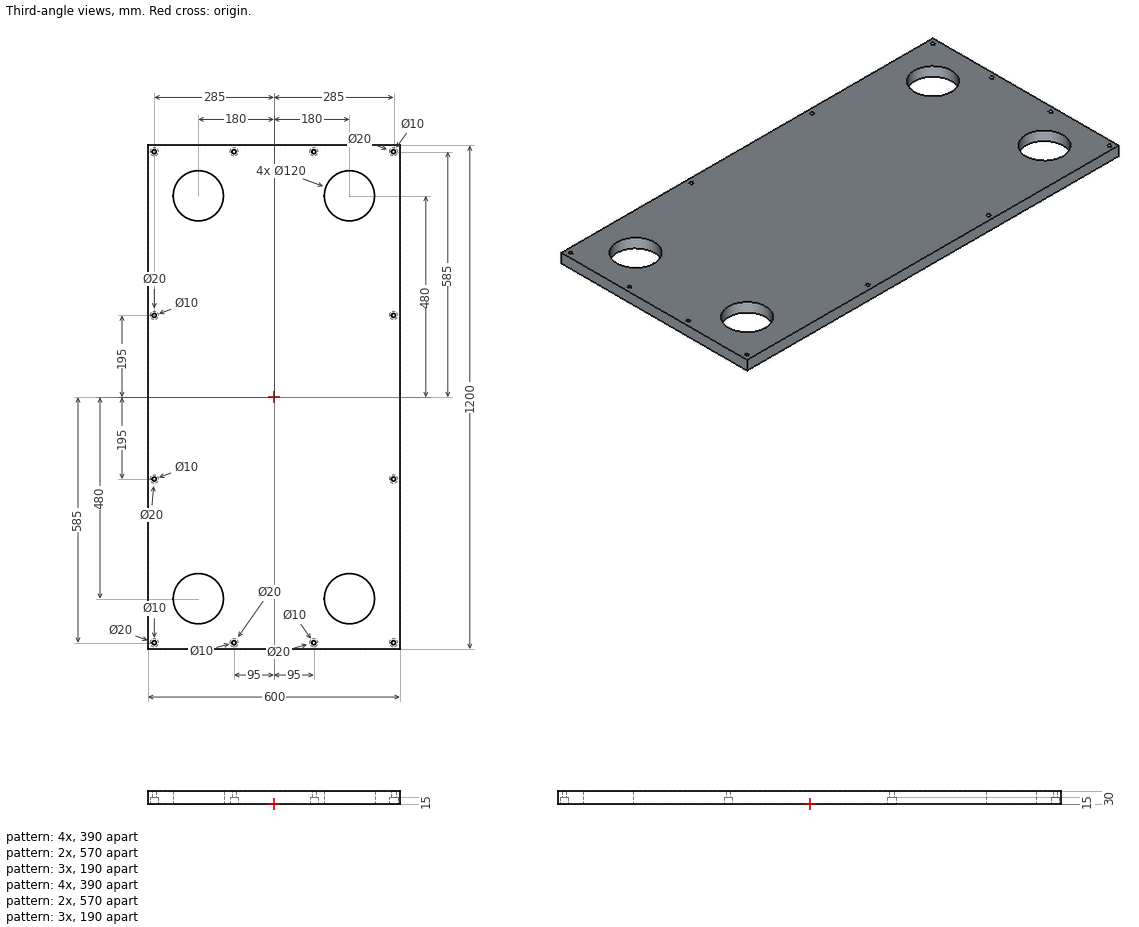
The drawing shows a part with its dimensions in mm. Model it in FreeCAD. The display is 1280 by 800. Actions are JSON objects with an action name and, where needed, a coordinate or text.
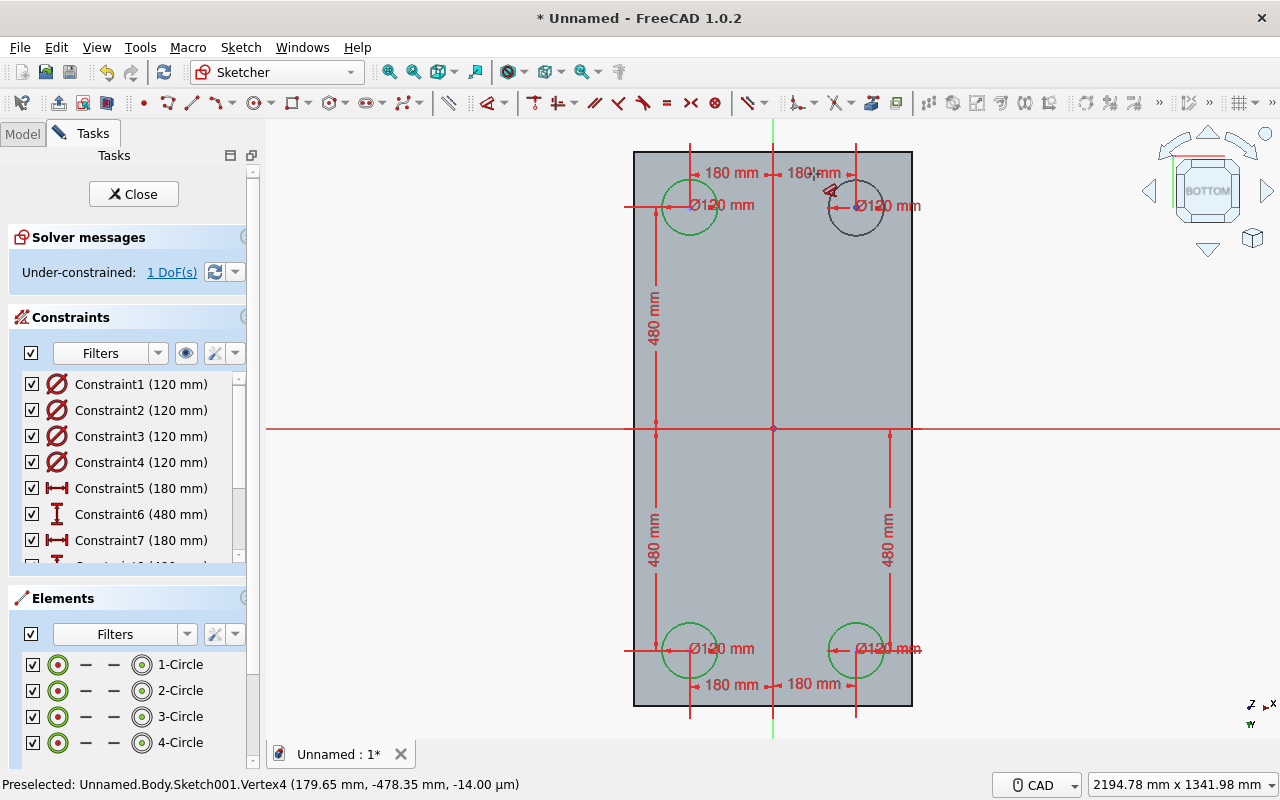
{"action": "left_click", "coordinate": [856, 208]}
{"action": "left_click", "coordinate": [890, 318]}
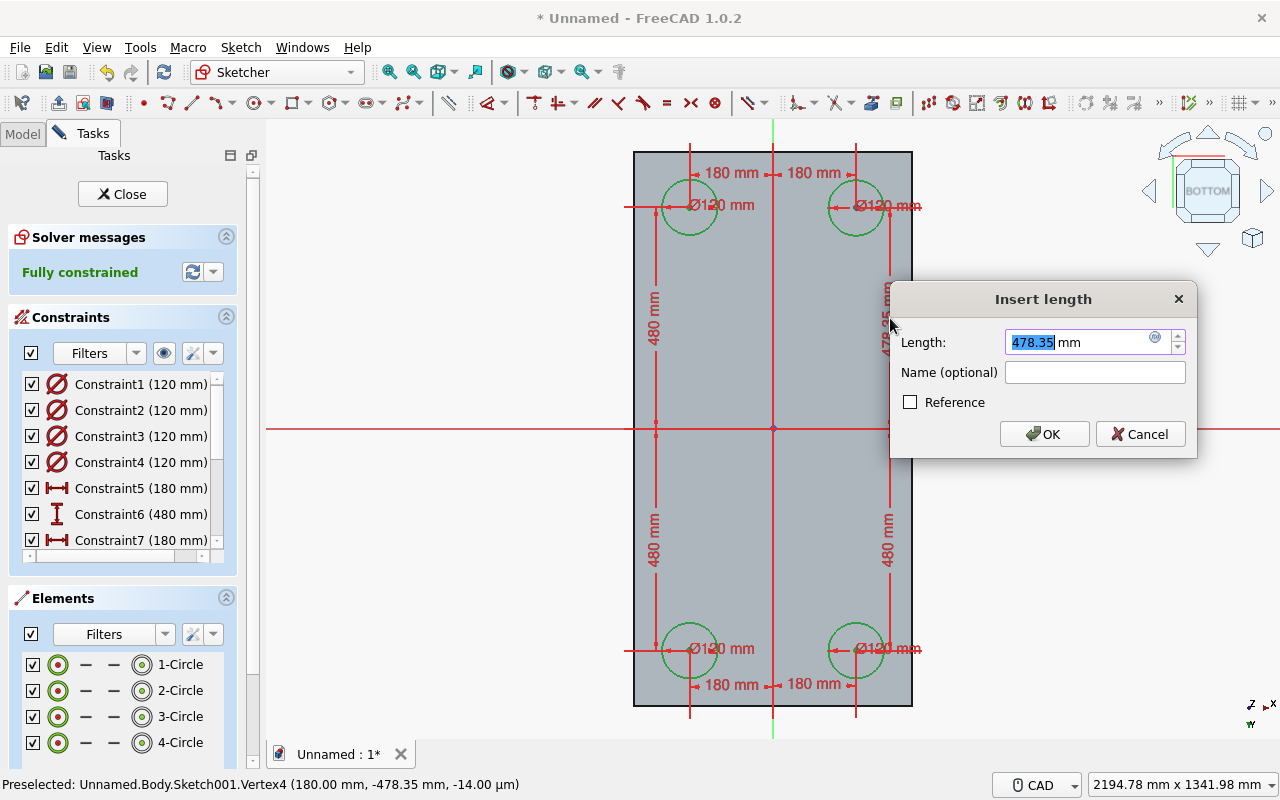
{"action": "type", "text": "480"}
{"action": "key", "text": "Return"}
{"action": "key", "text": "Escape"}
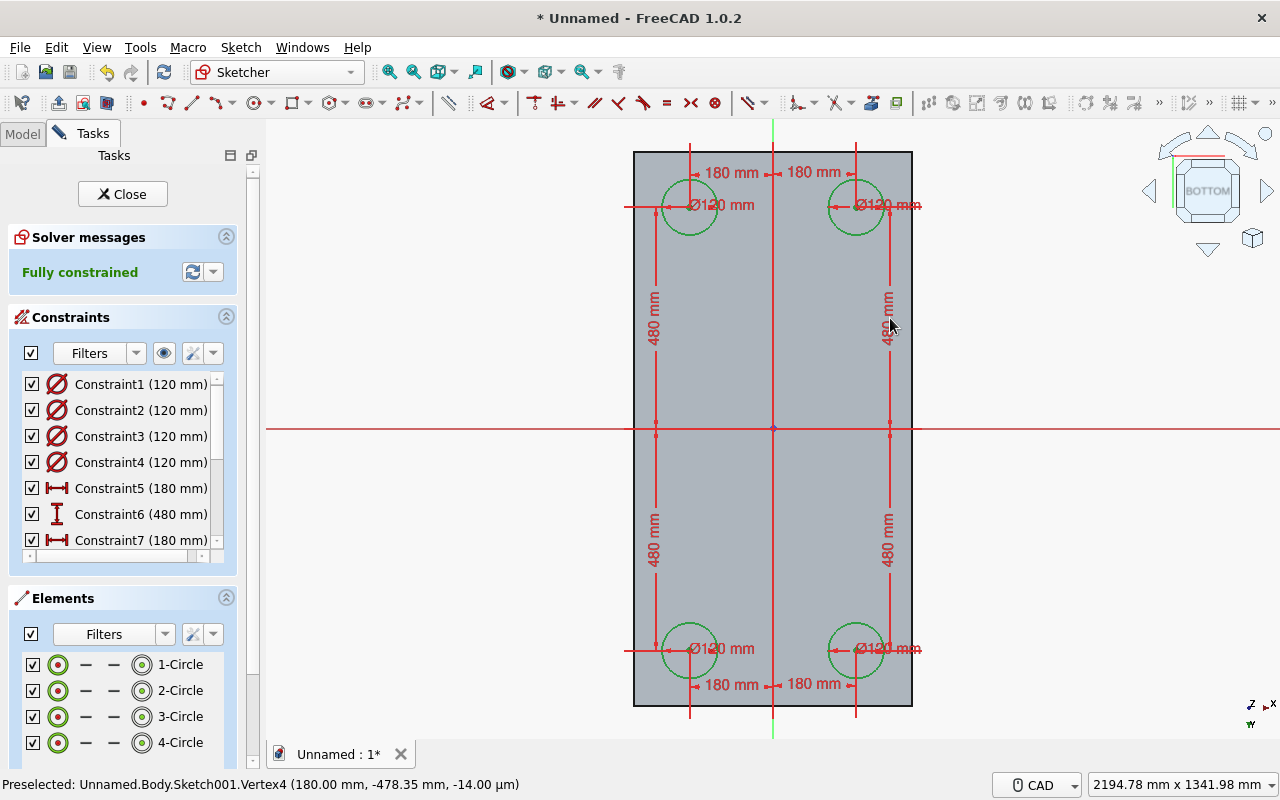
{"action": "left_click", "coordinate": [123, 194]}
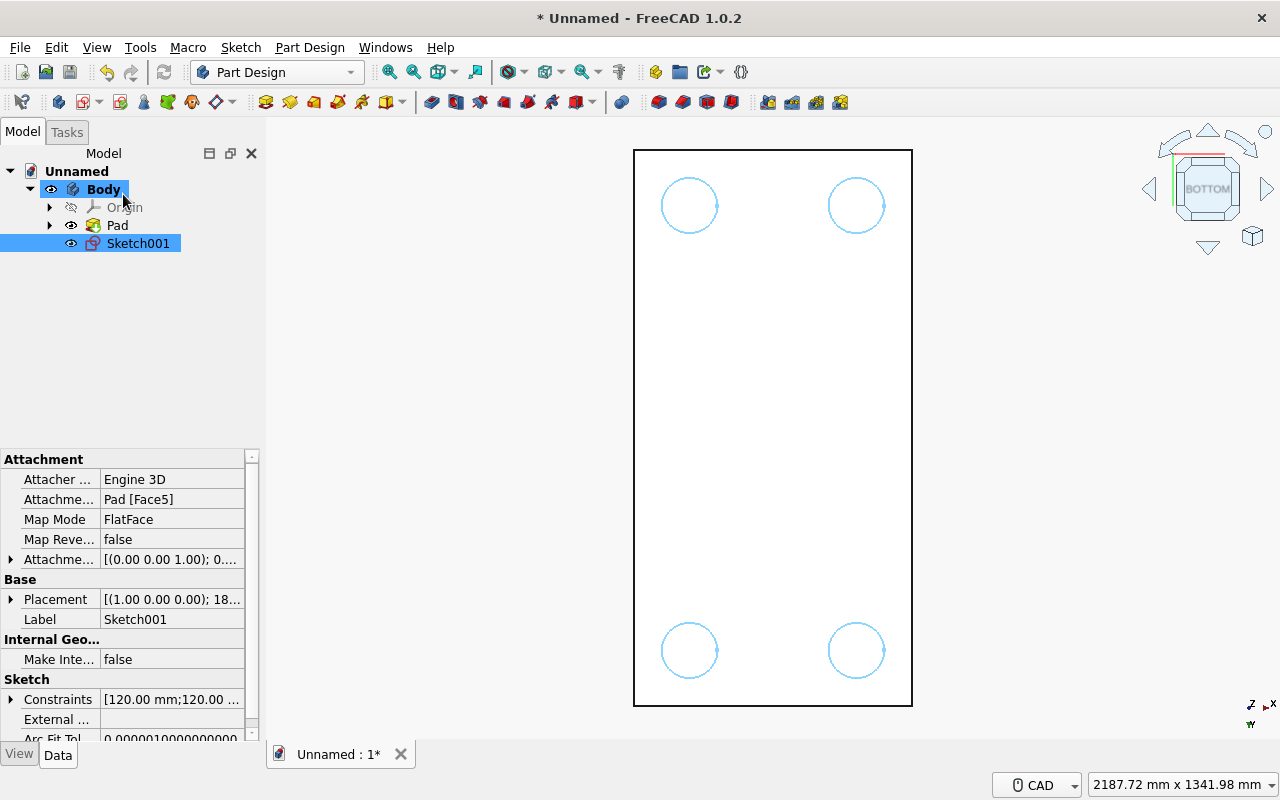
{"action": "left_click", "coordinate": [432, 102]}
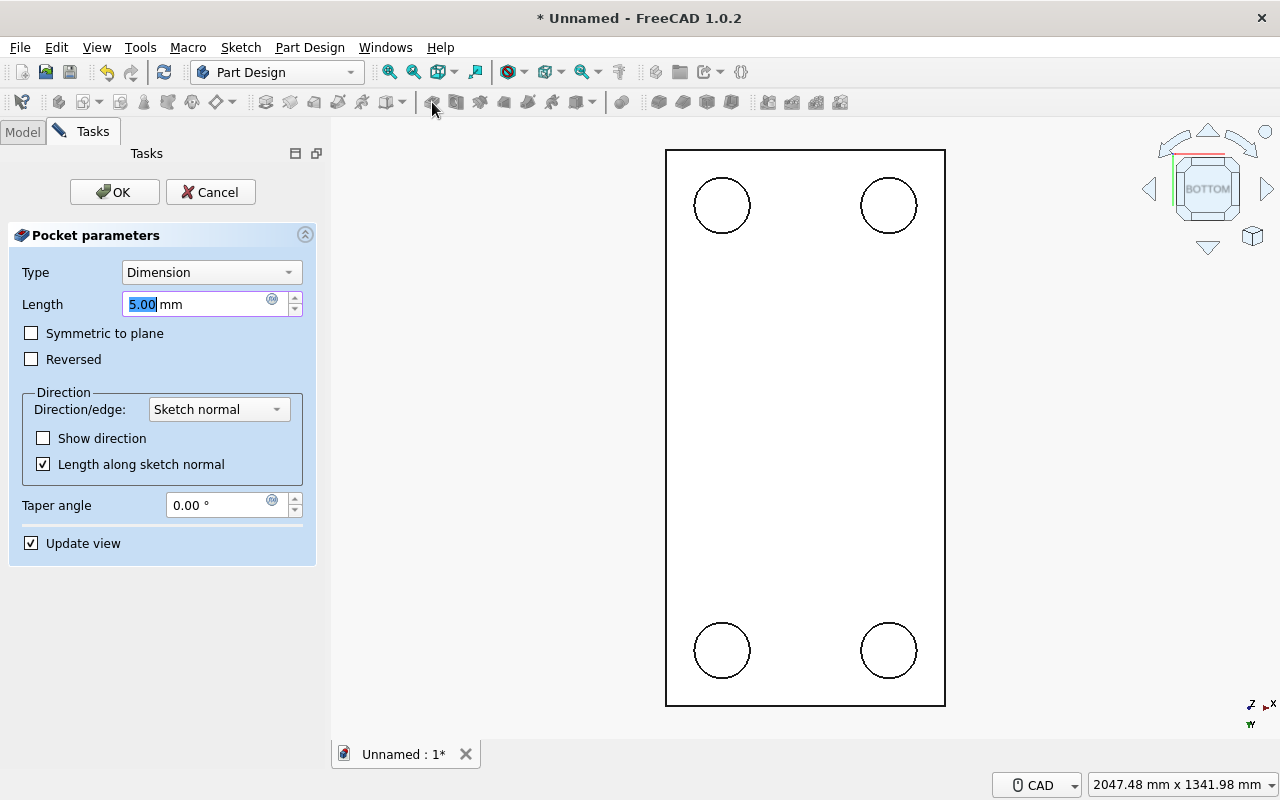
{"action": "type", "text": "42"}
{"action": "key", "text": "Tab"}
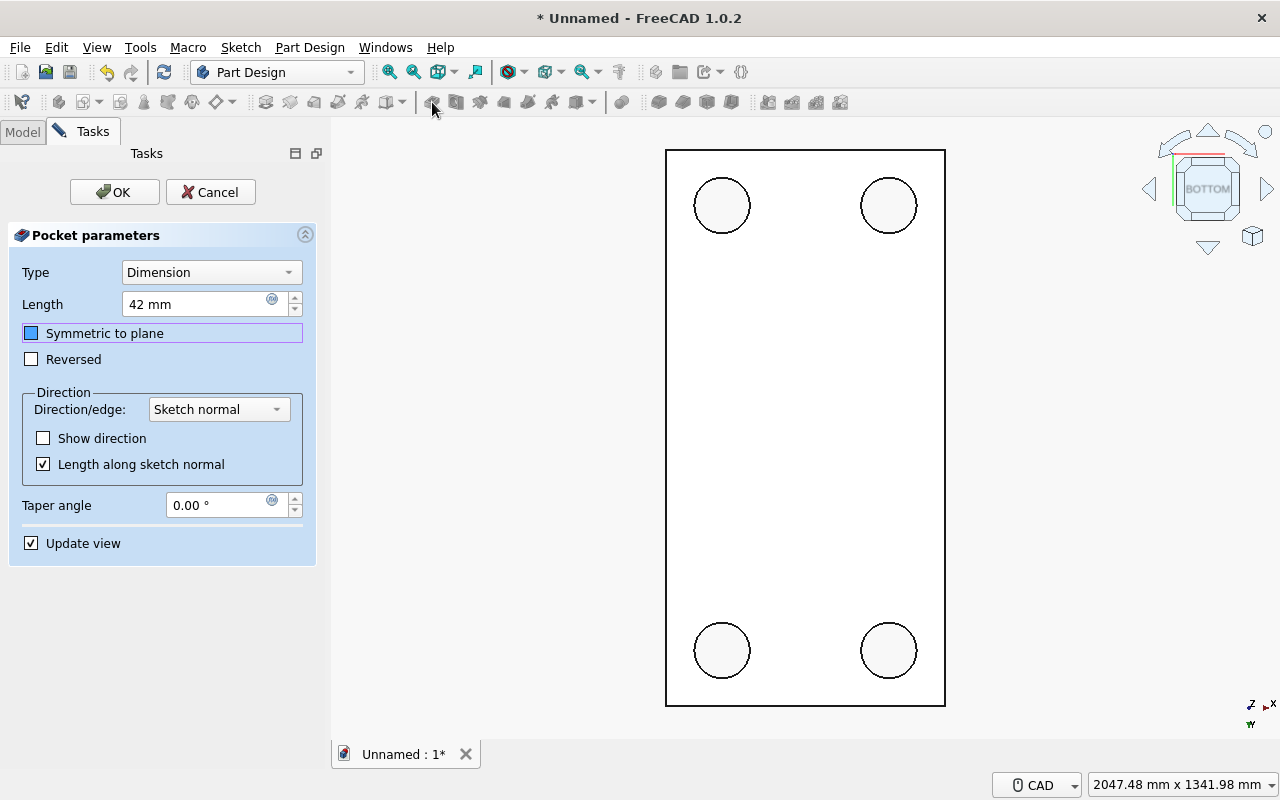
{"action": "left_click", "coordinate": [115, 192]}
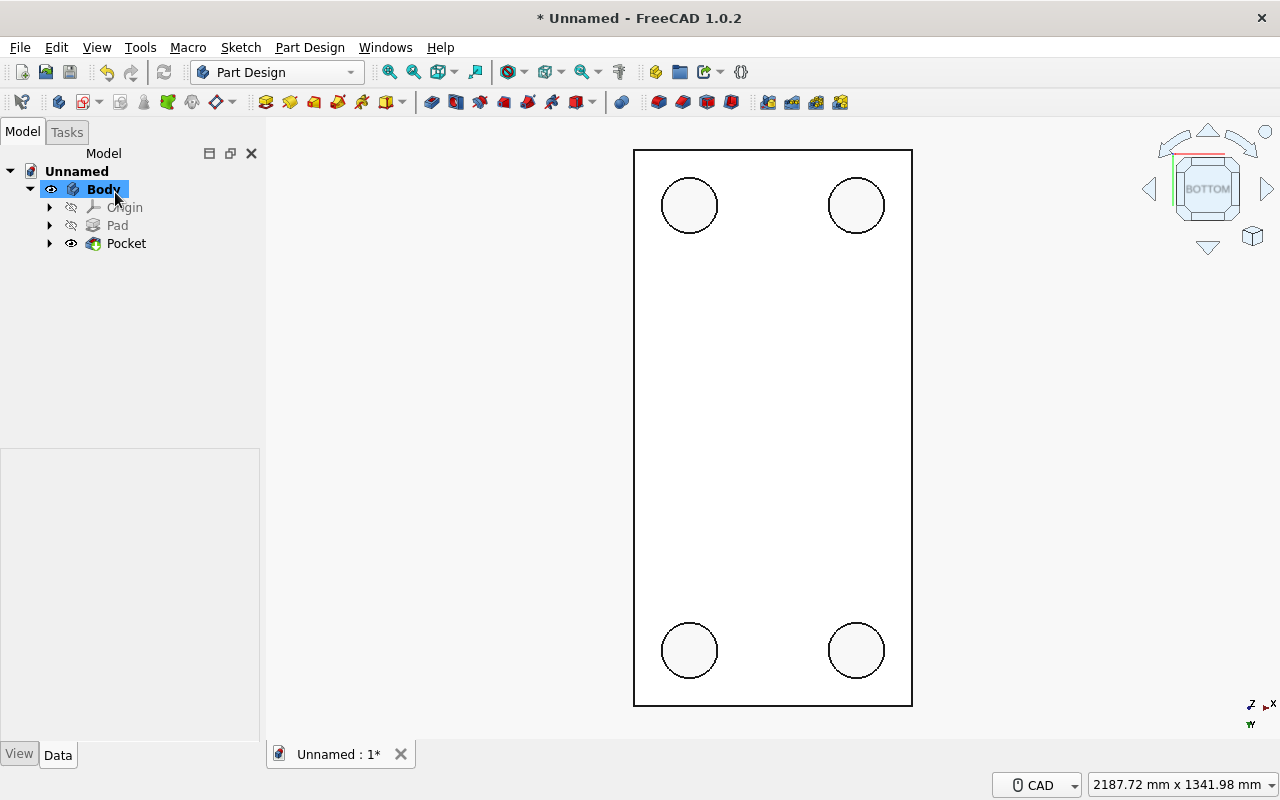
{"action": "left_click", "coordinate": [84, 102]}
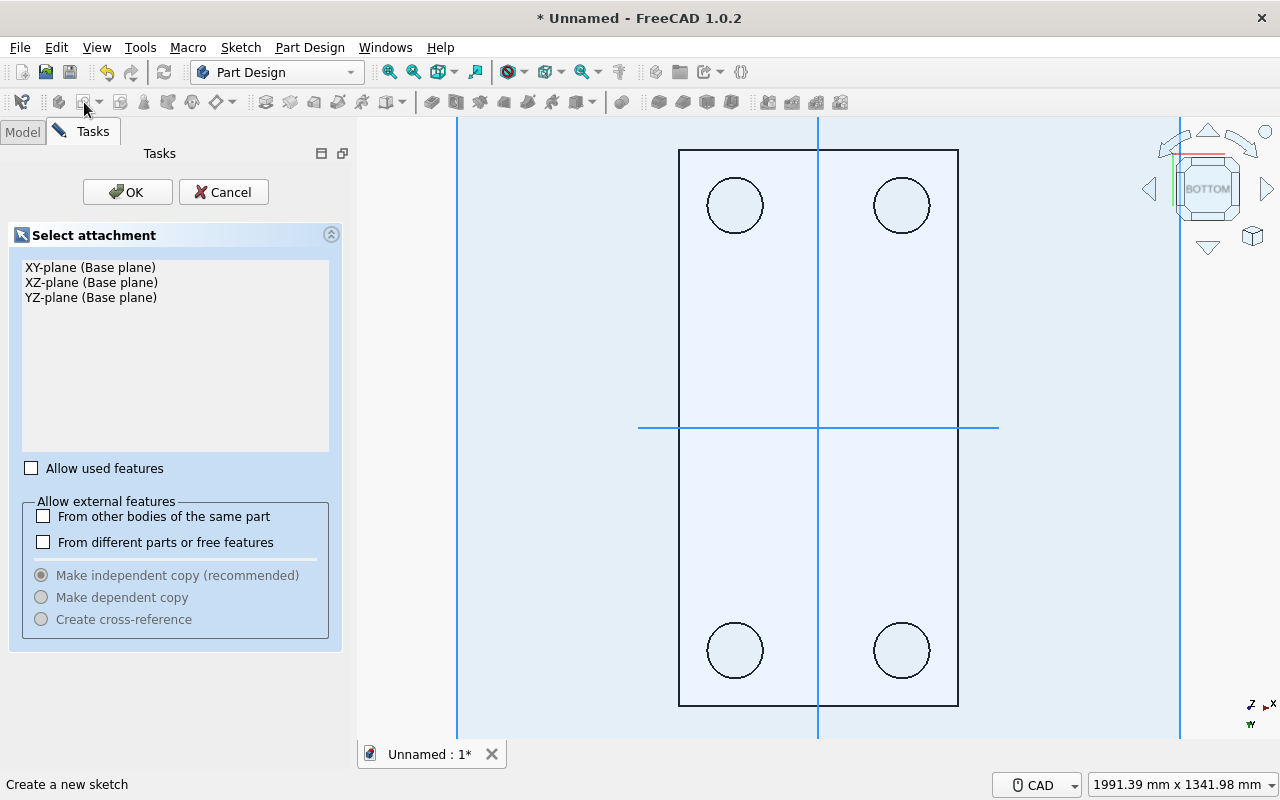
{"action": "left_click", "coordinate": [82, 268]}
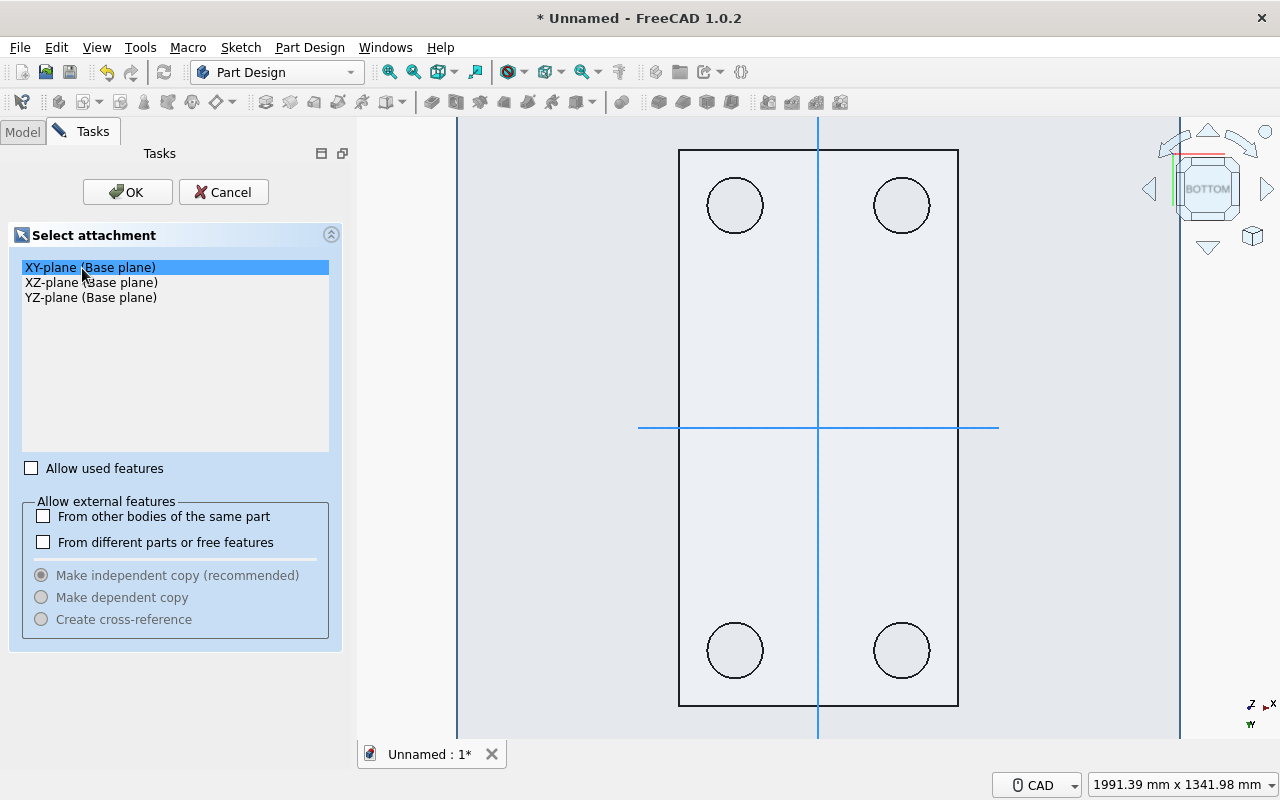
{"action": "left_click", "coordinate": [128, 192]}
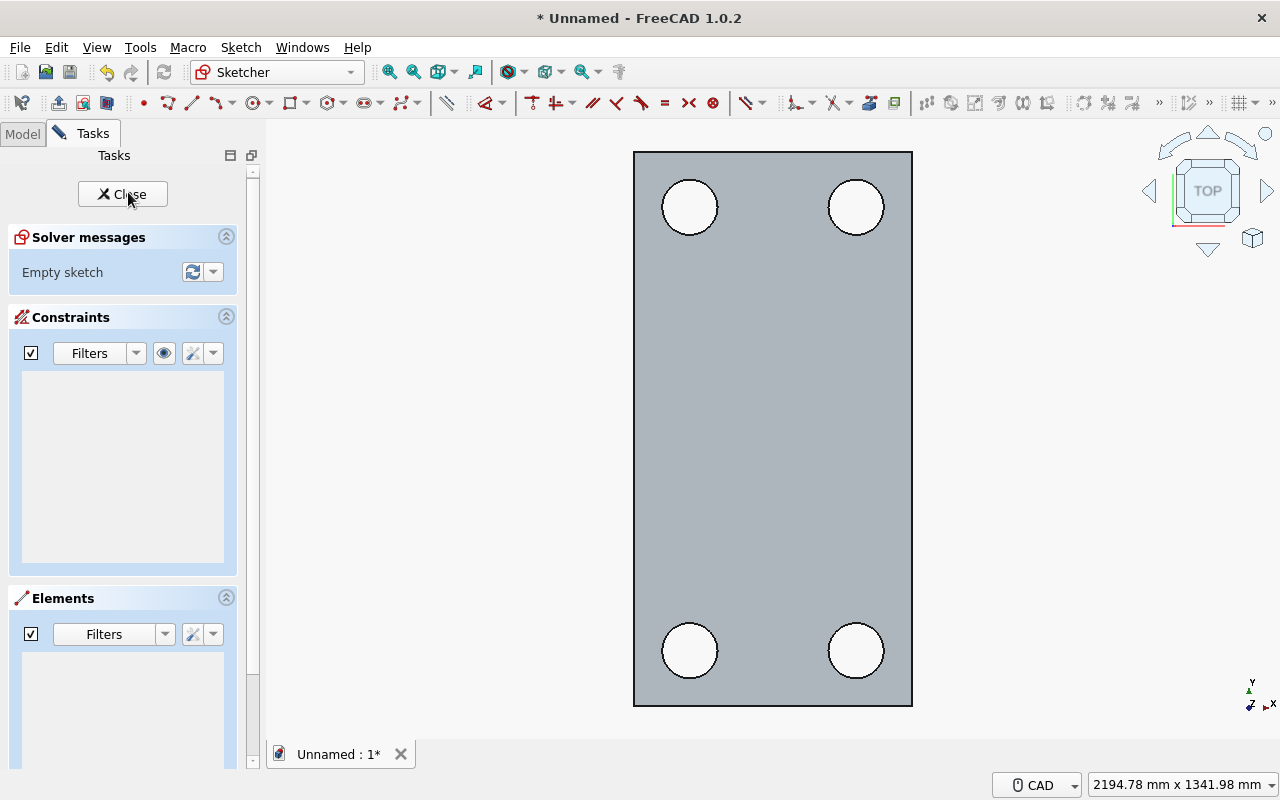
{"action": "left_click", "coordinate": [108, 104]}